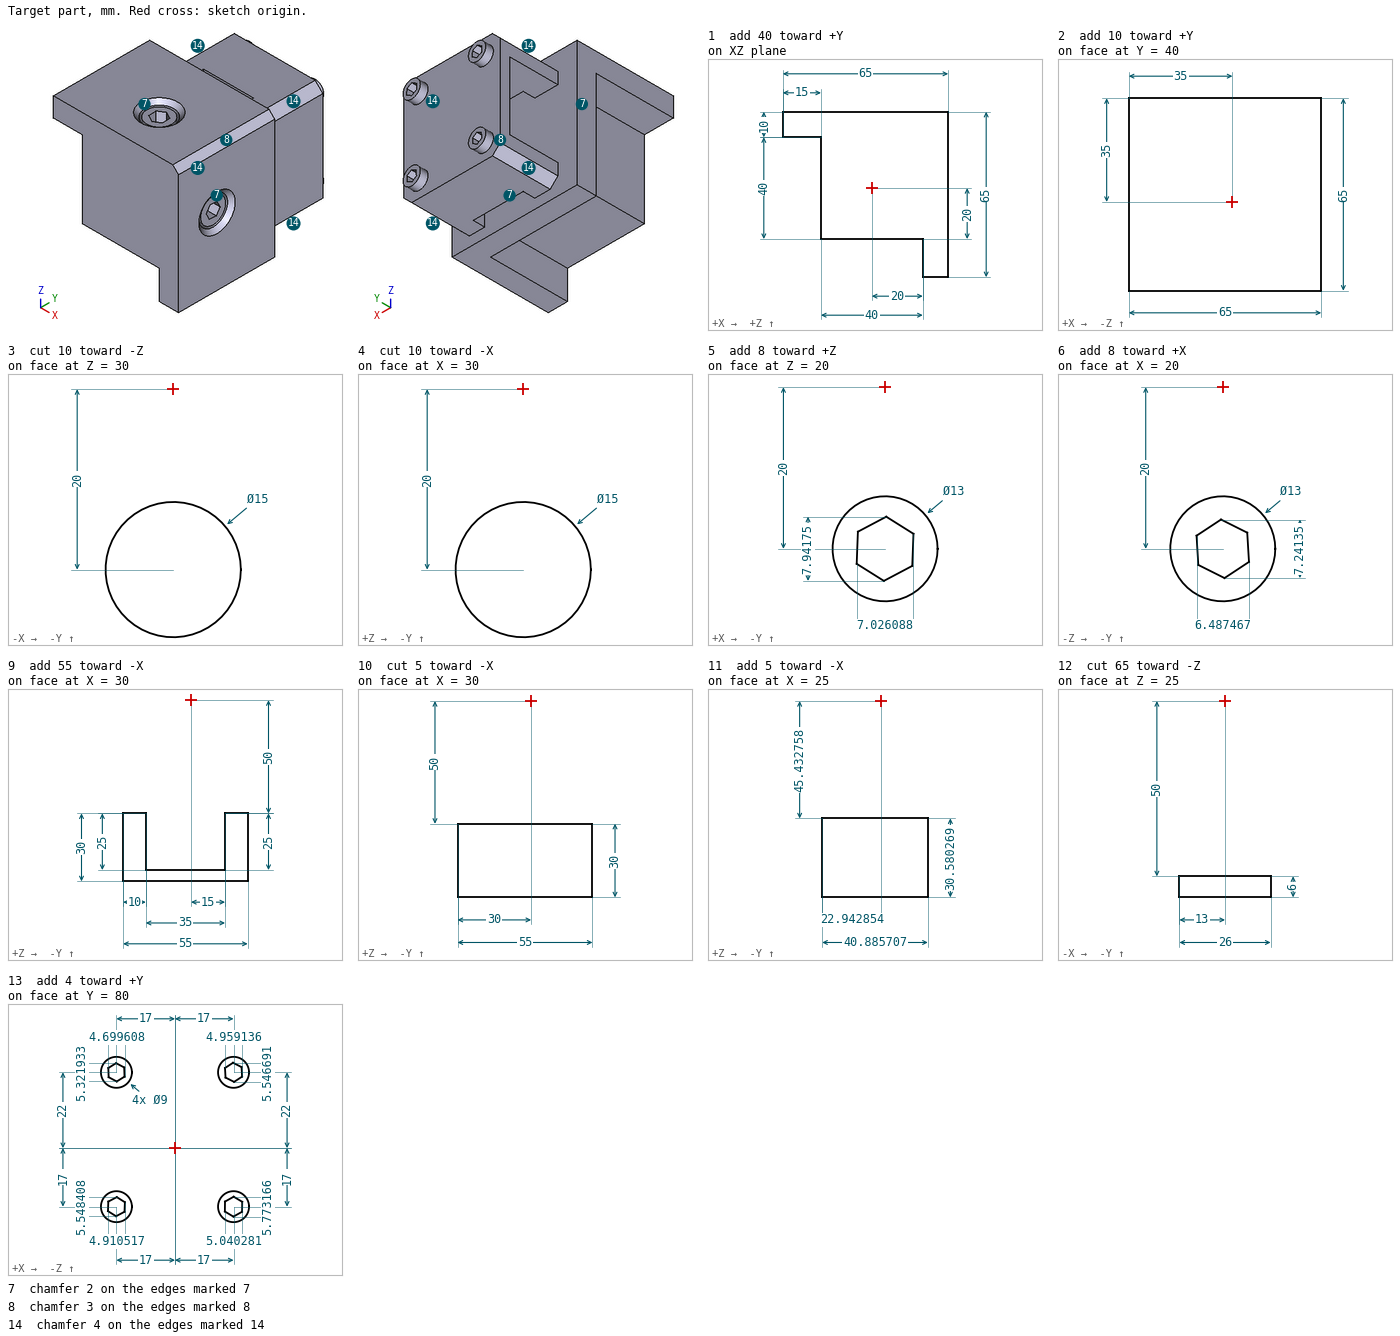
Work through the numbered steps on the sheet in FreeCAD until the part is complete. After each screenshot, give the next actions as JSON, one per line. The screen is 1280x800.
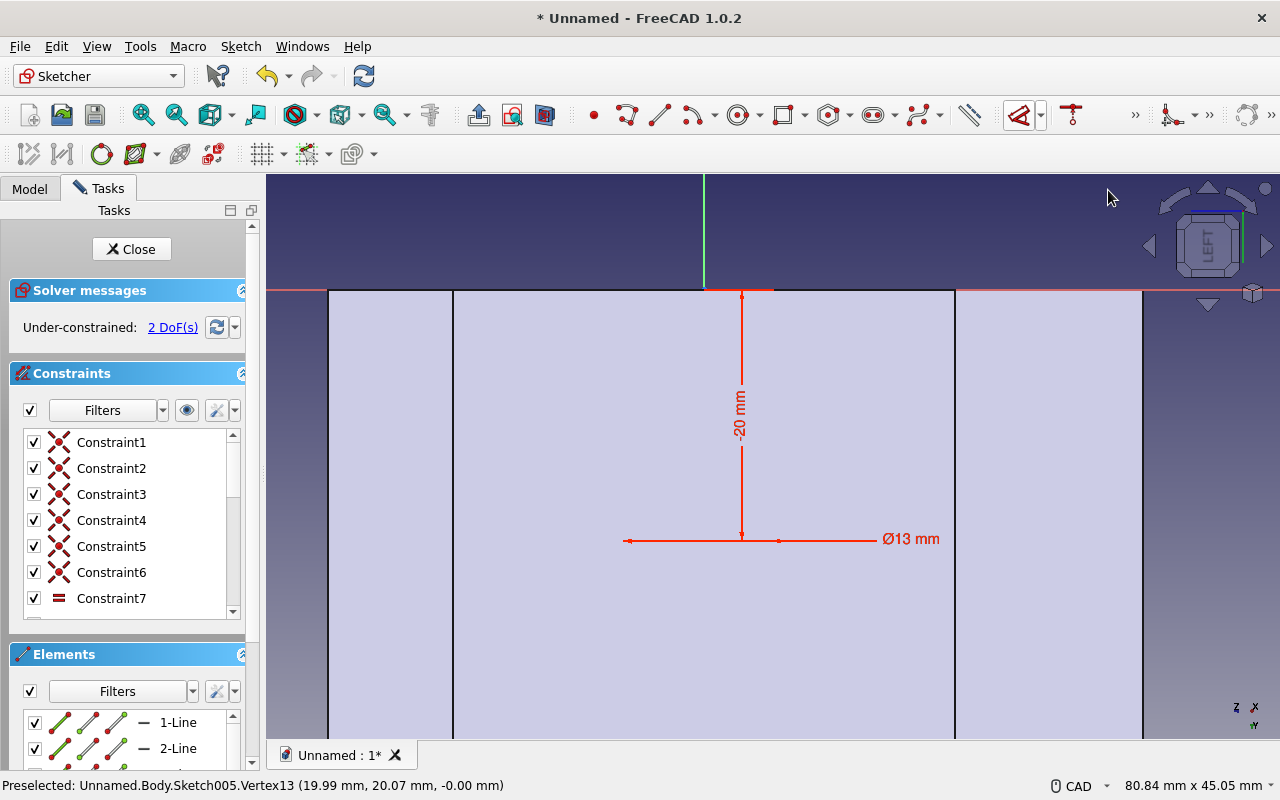
{"action": "left_click", "coordinate": [663, 522]}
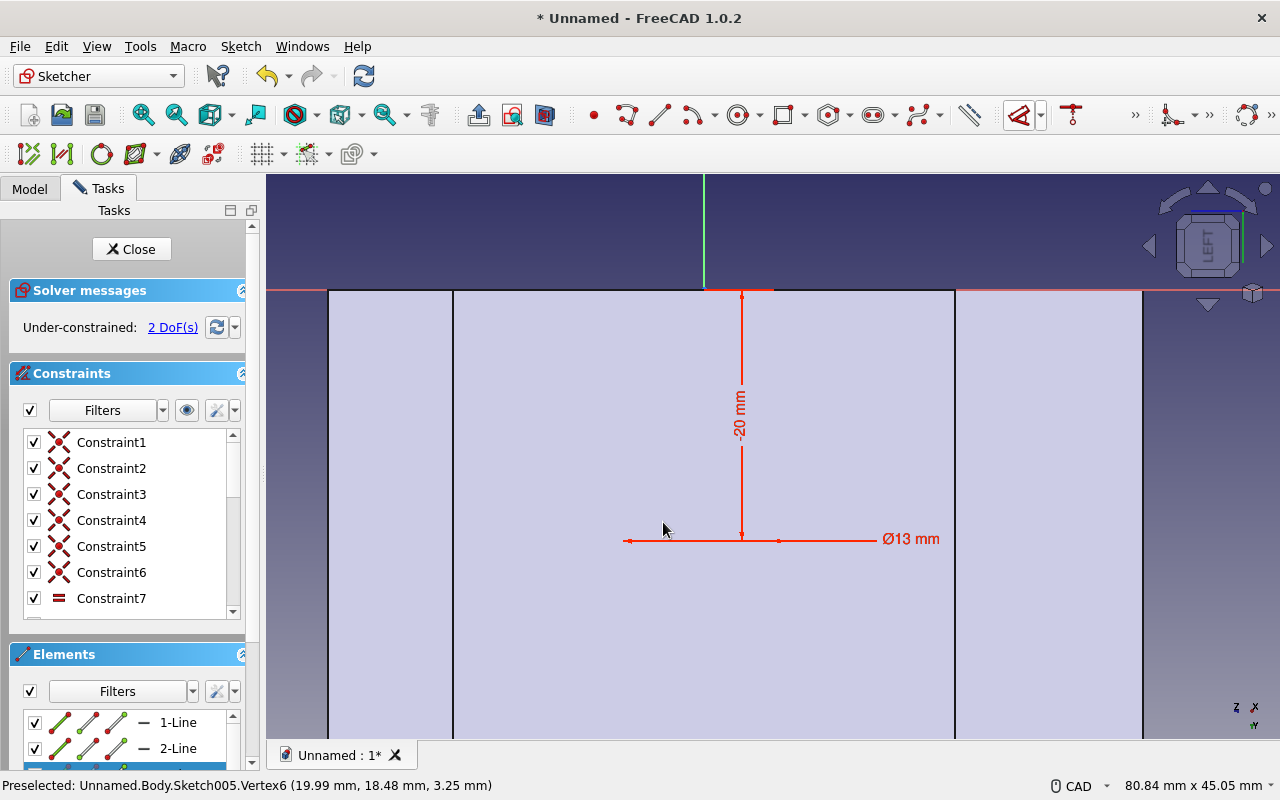
{"action": "left_click", "coordinate": [745, 560]}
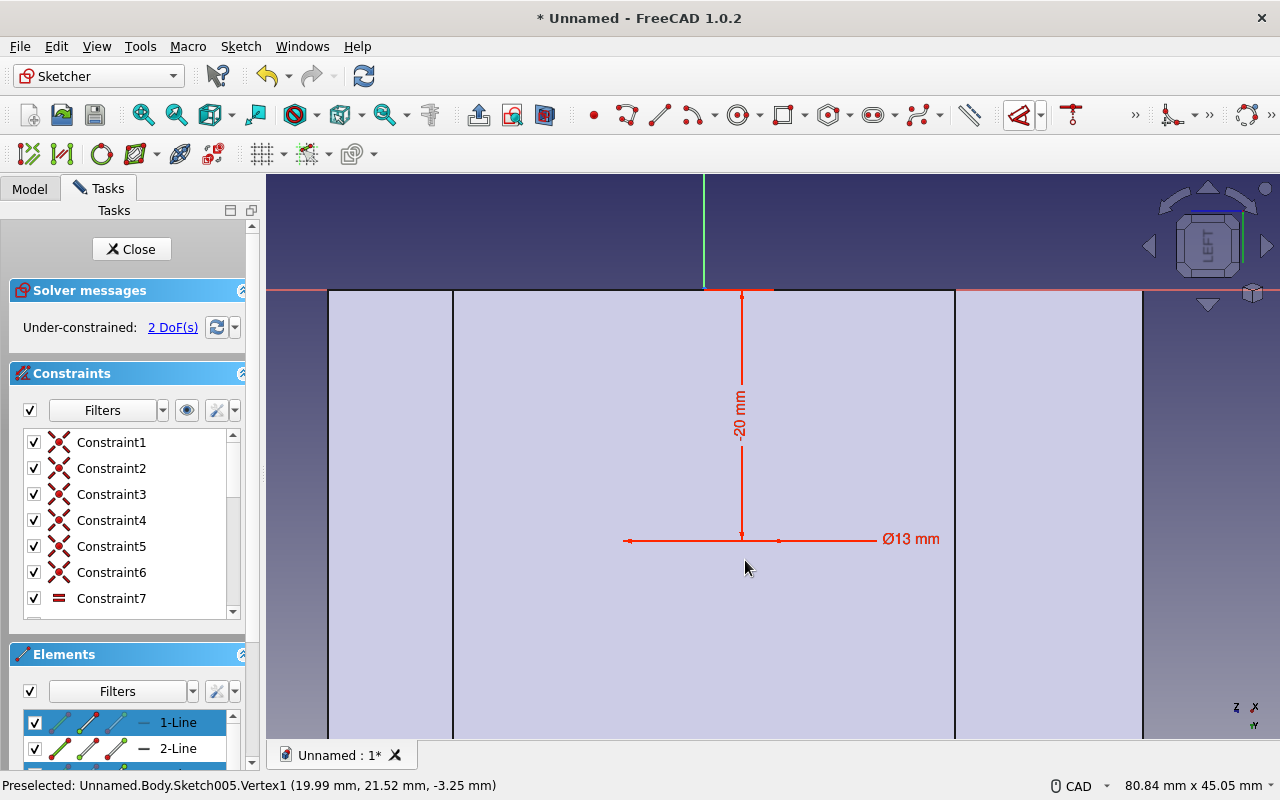
{"action": "left_click", "coordinate": [1040, 116]}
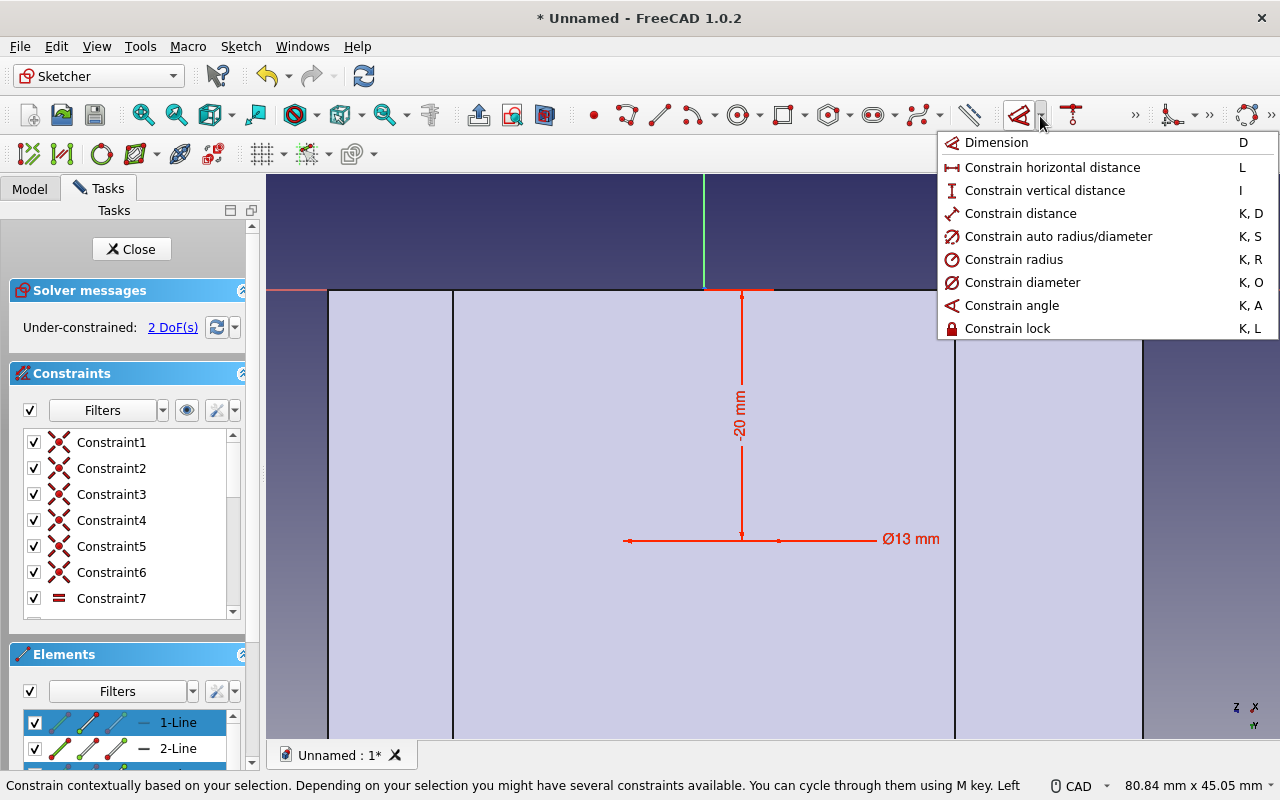
{"action": "left_click", "coordinate": [1108, 168]}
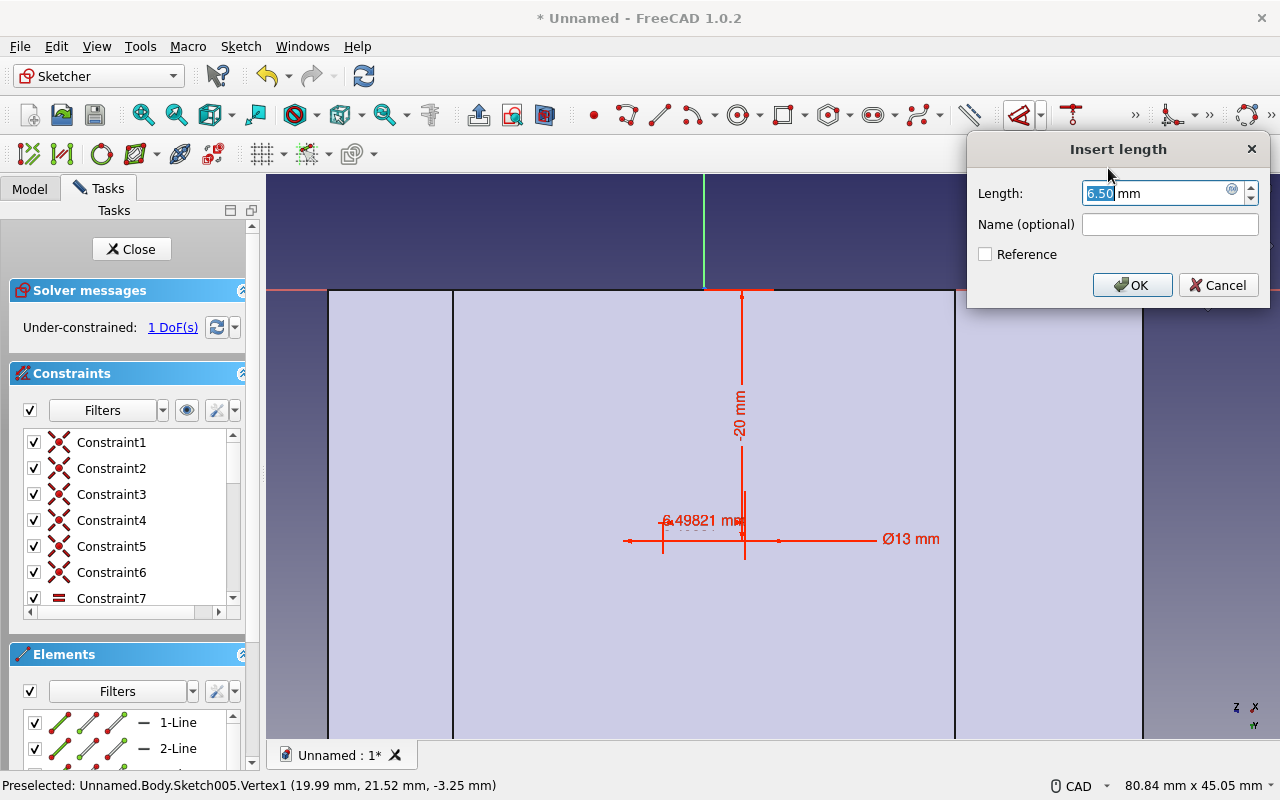
{"action": "type", "text": "6.487467"}
{"action": "key", "text": "Return"}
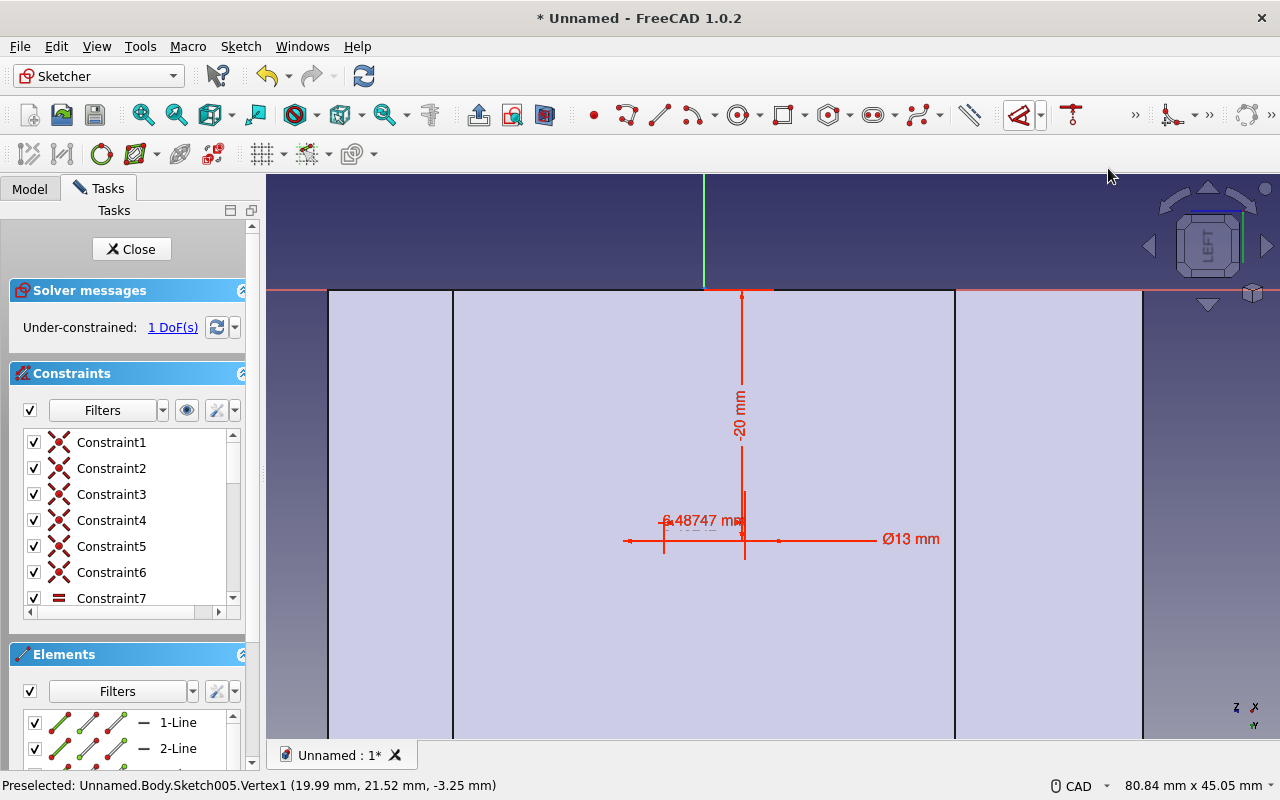
{"action": "left_click", "coordinate": [708, 586]}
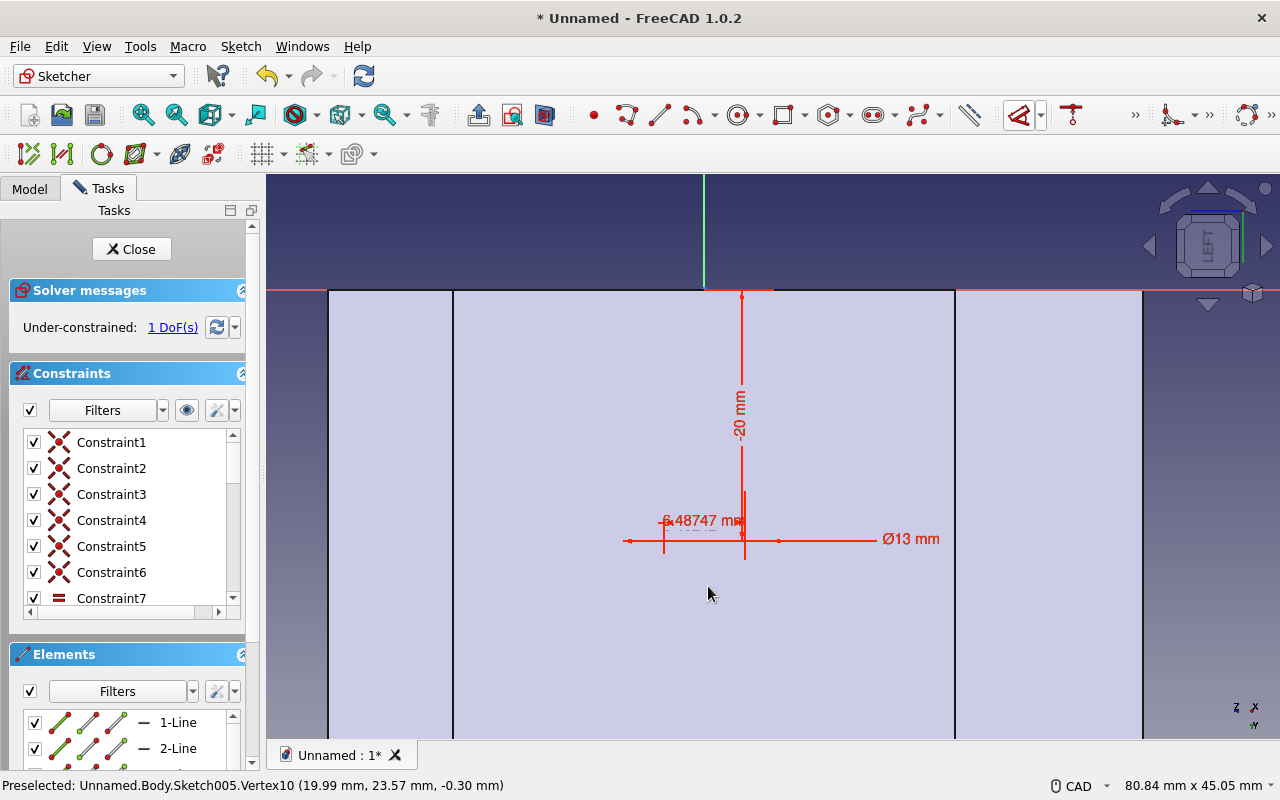
{"action": "left_click", "coordinate": [700, 496]}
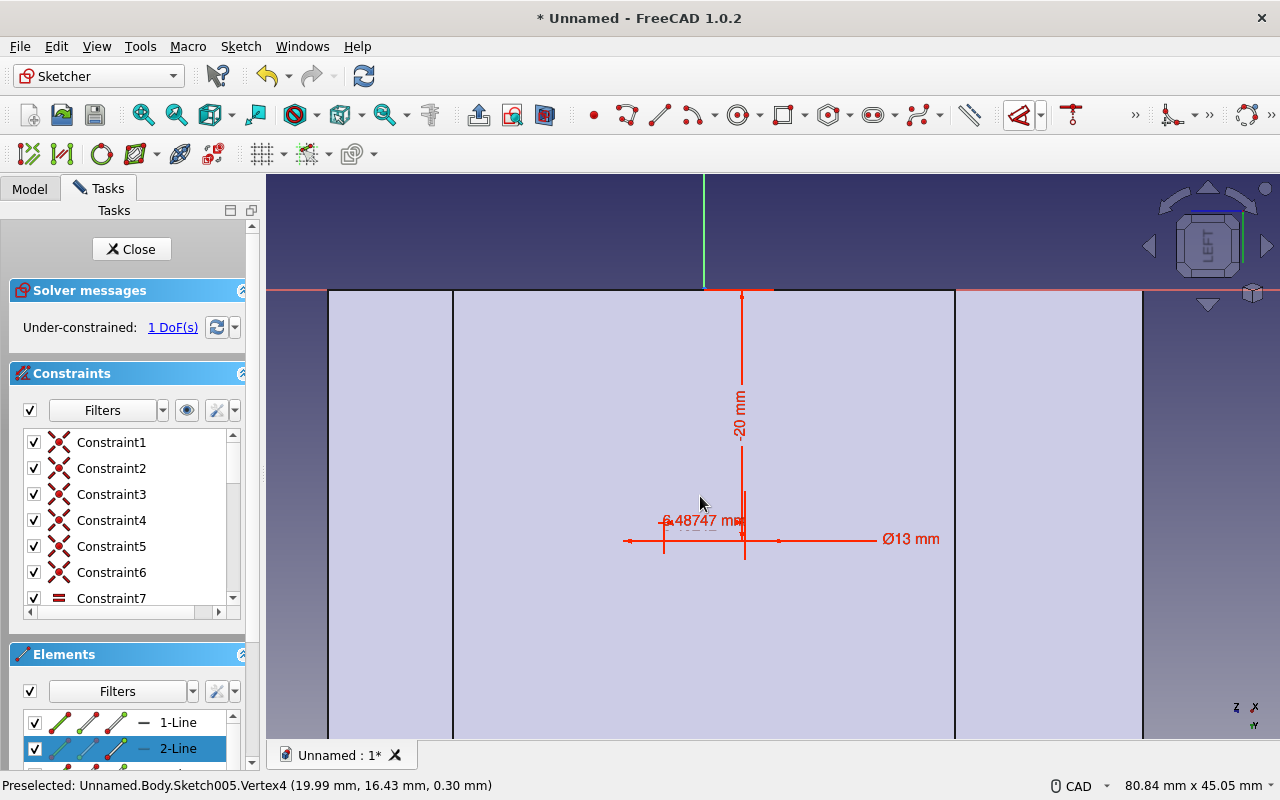
{"action": "left_click", "coordinate": [1040, 116]}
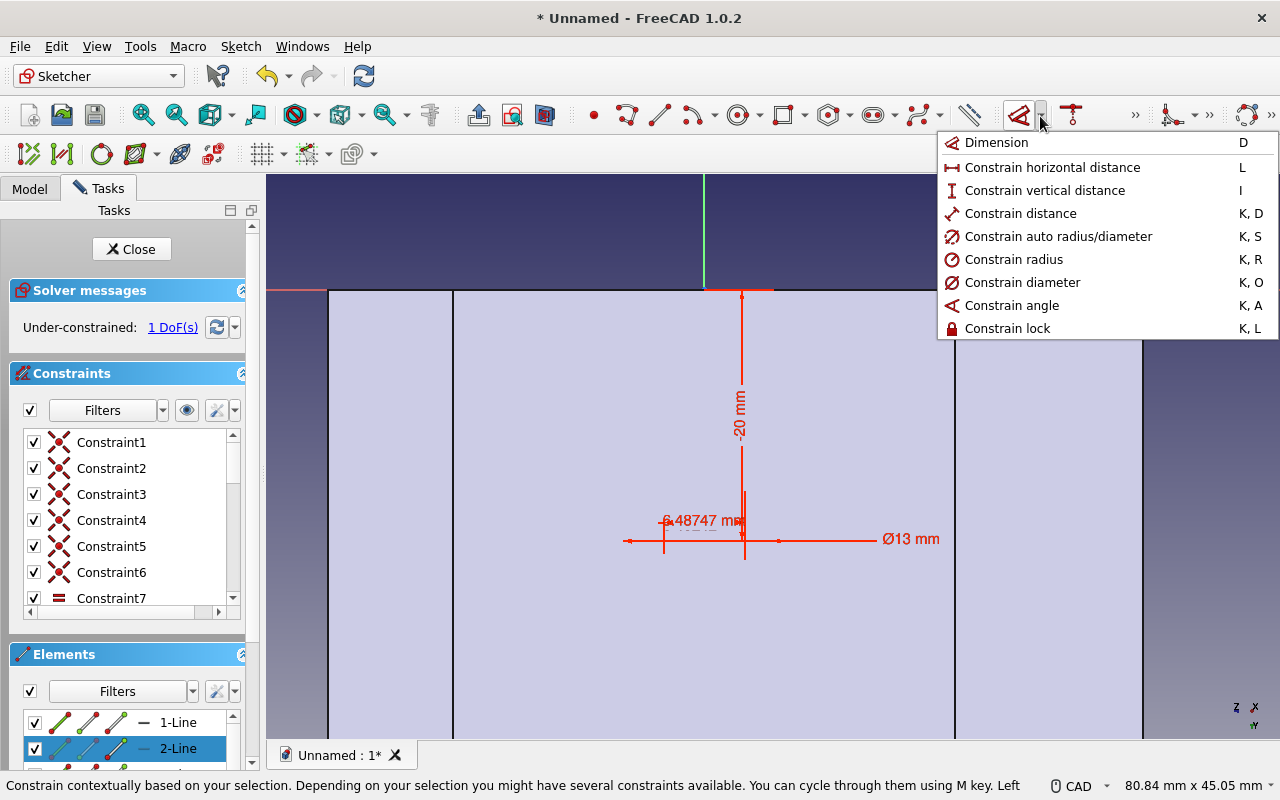
{"action": "left_click", "coordinate": [1108, 190]}